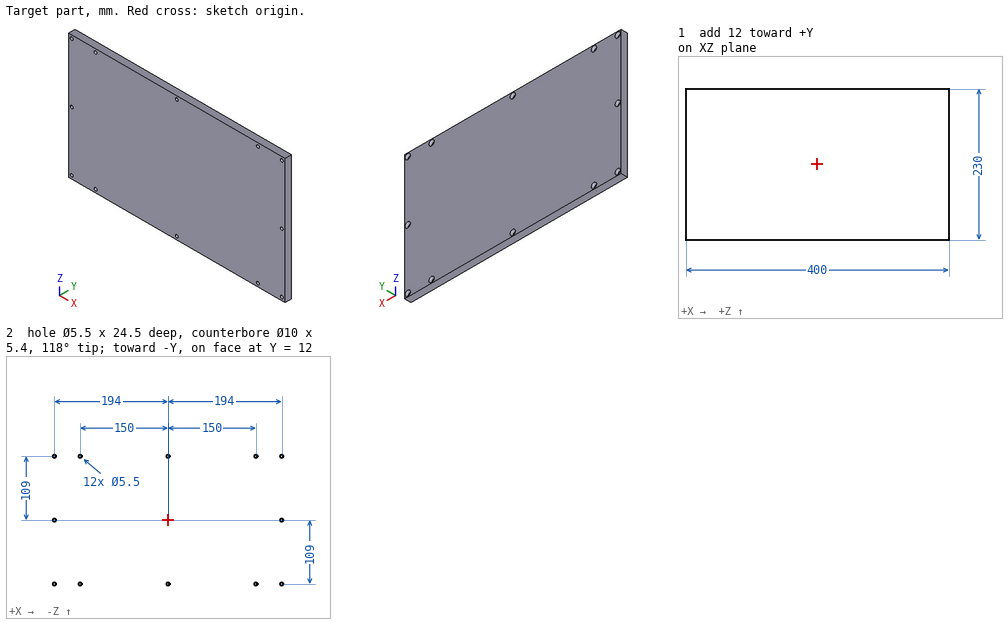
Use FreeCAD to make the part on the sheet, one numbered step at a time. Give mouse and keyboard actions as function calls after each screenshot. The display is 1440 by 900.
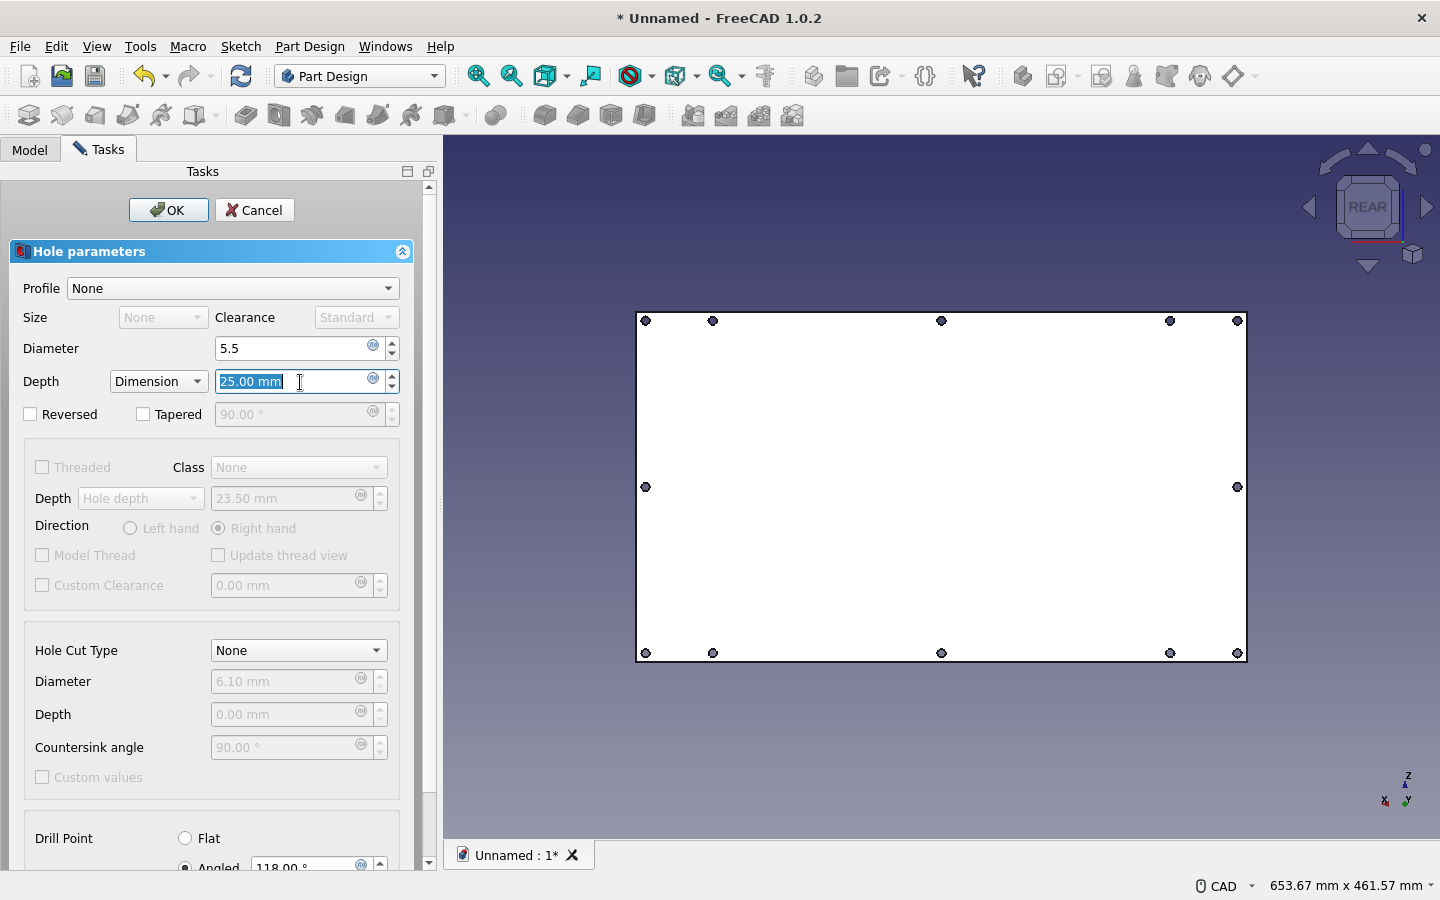
text(24.5)
key(Tab)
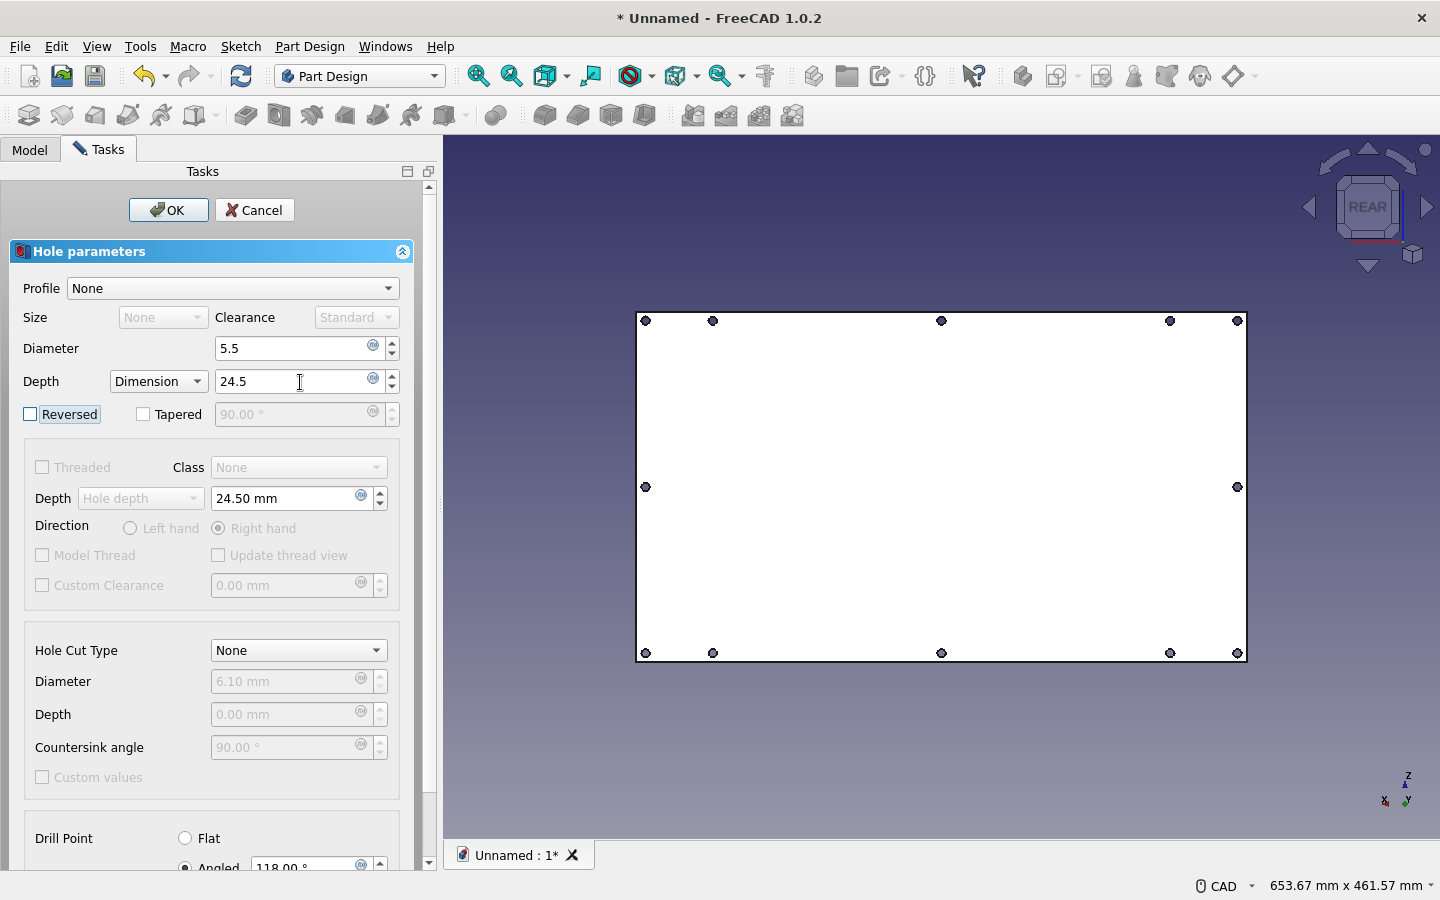
click(300, 650)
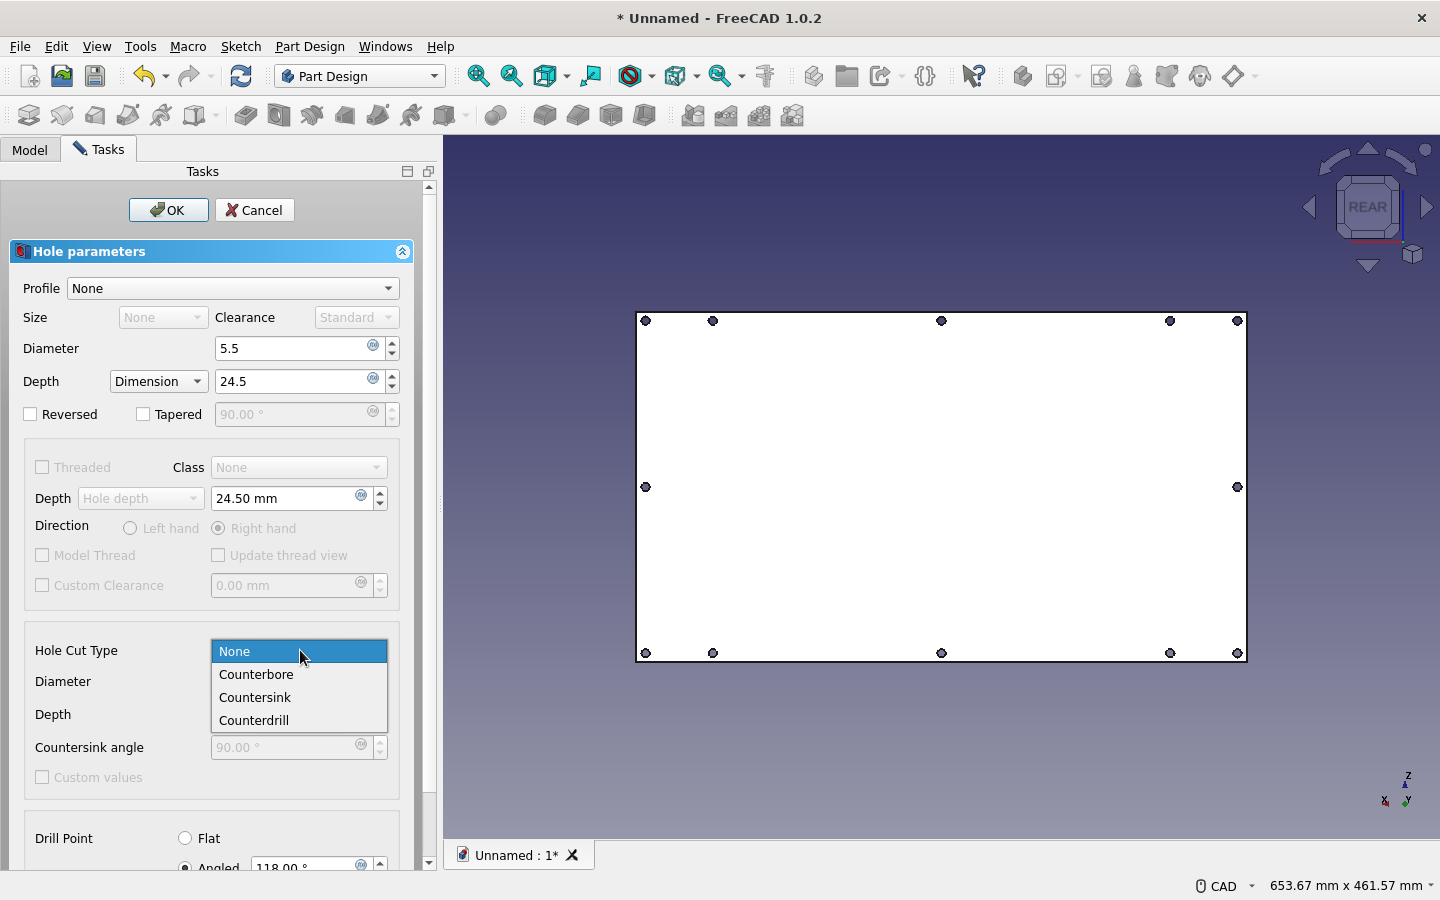
click(298, 674)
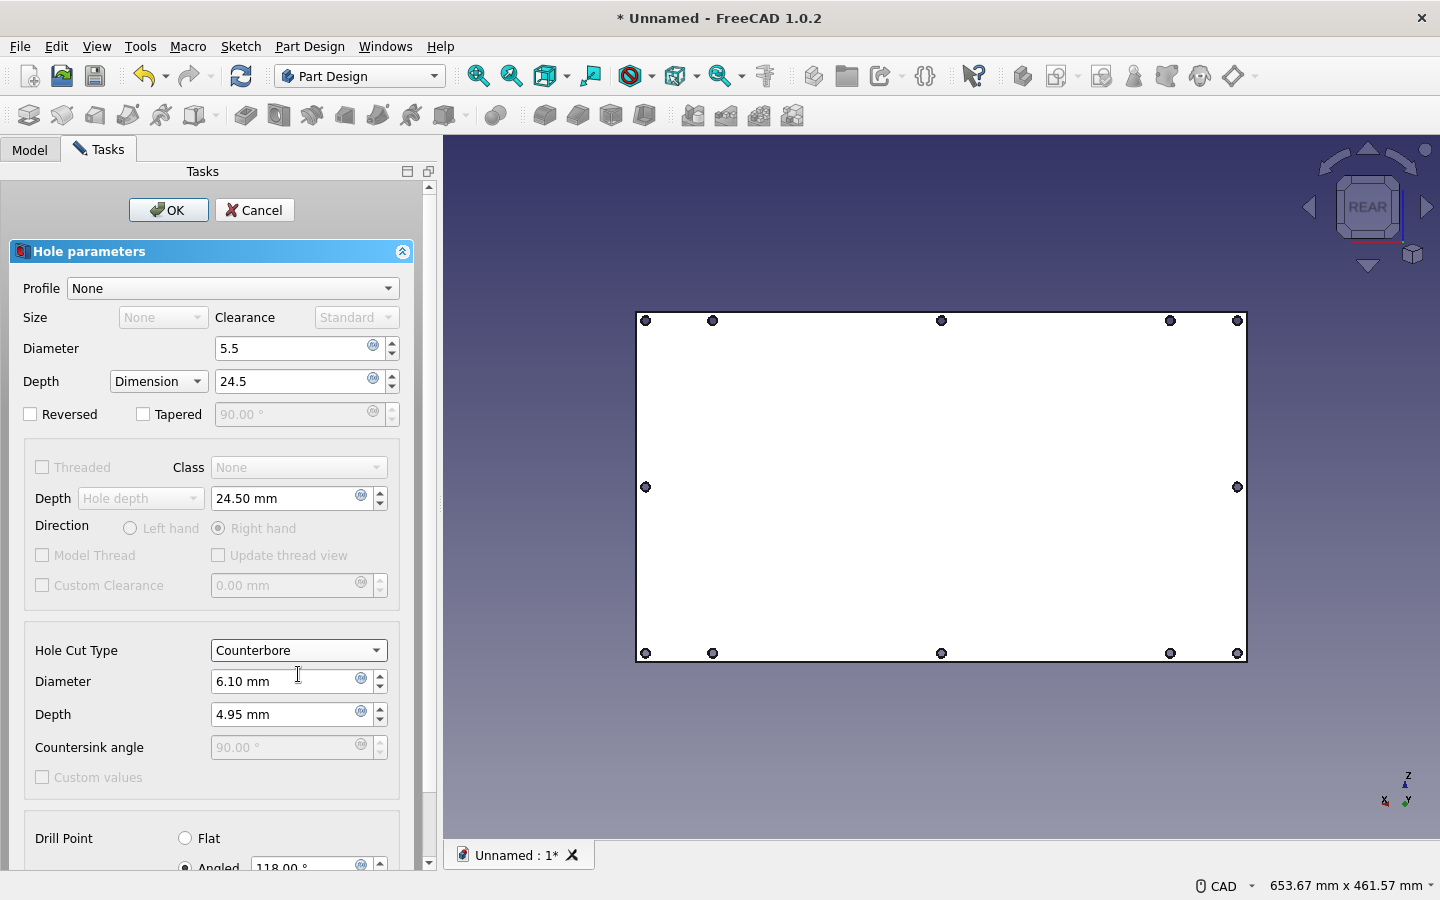
triple_click(292, 682)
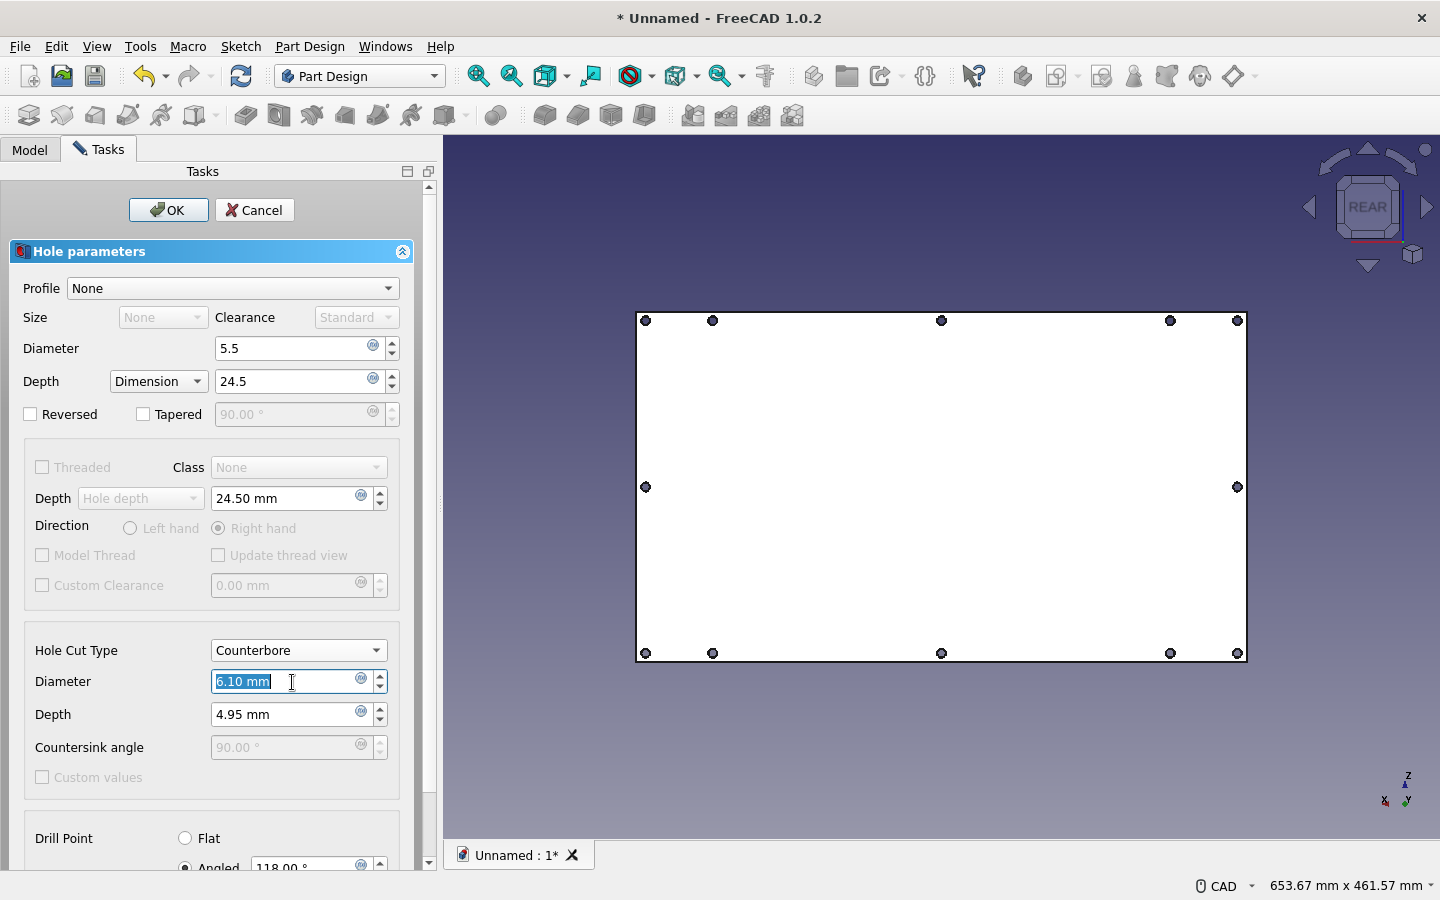
text(10)
key(Tab)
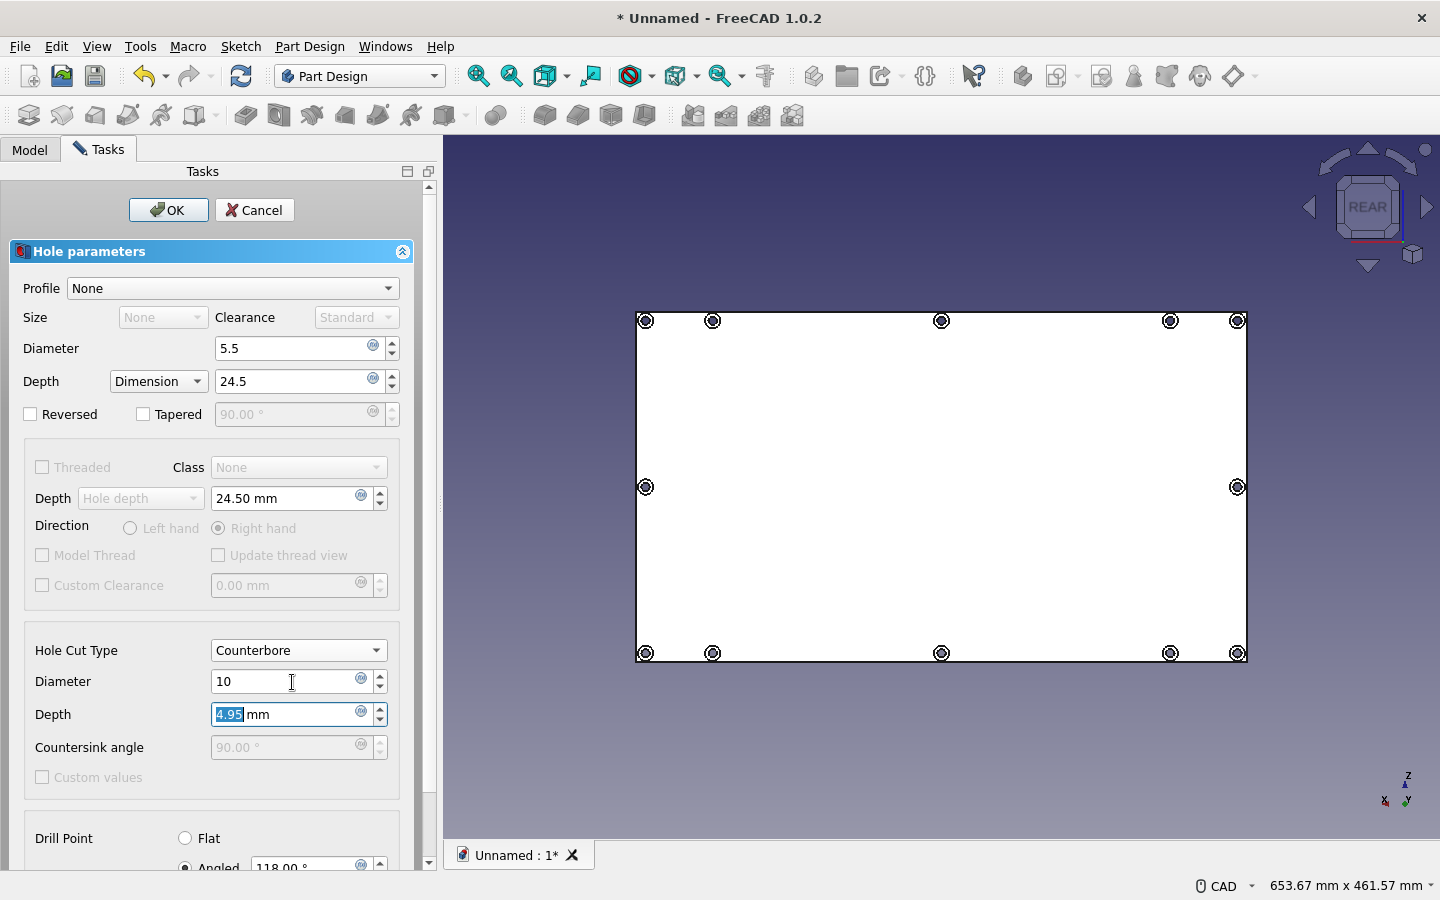
text(5.4)
key(Tab)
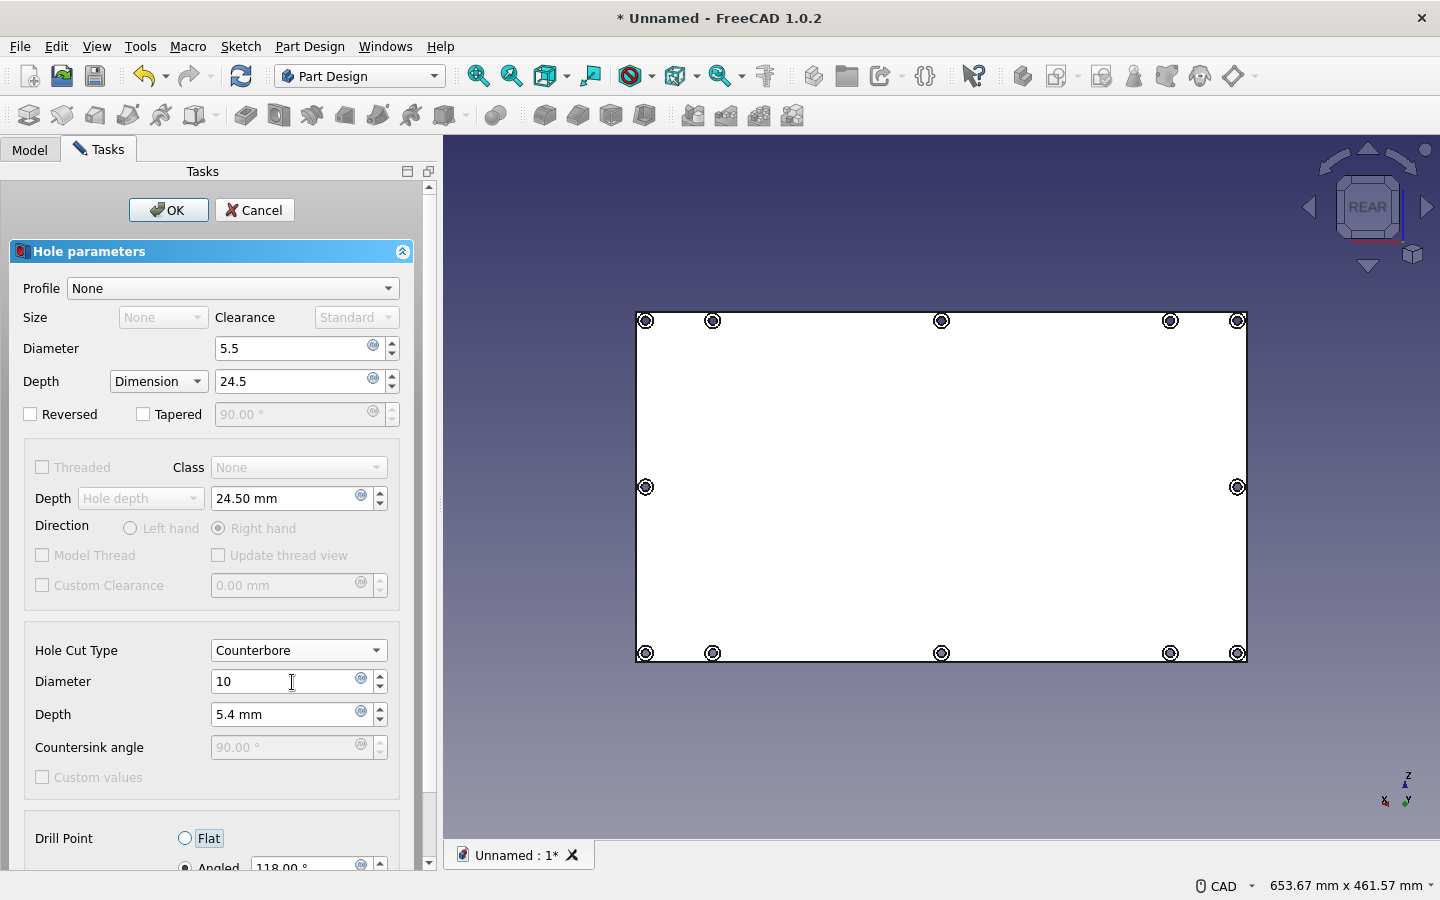
click(169, 210)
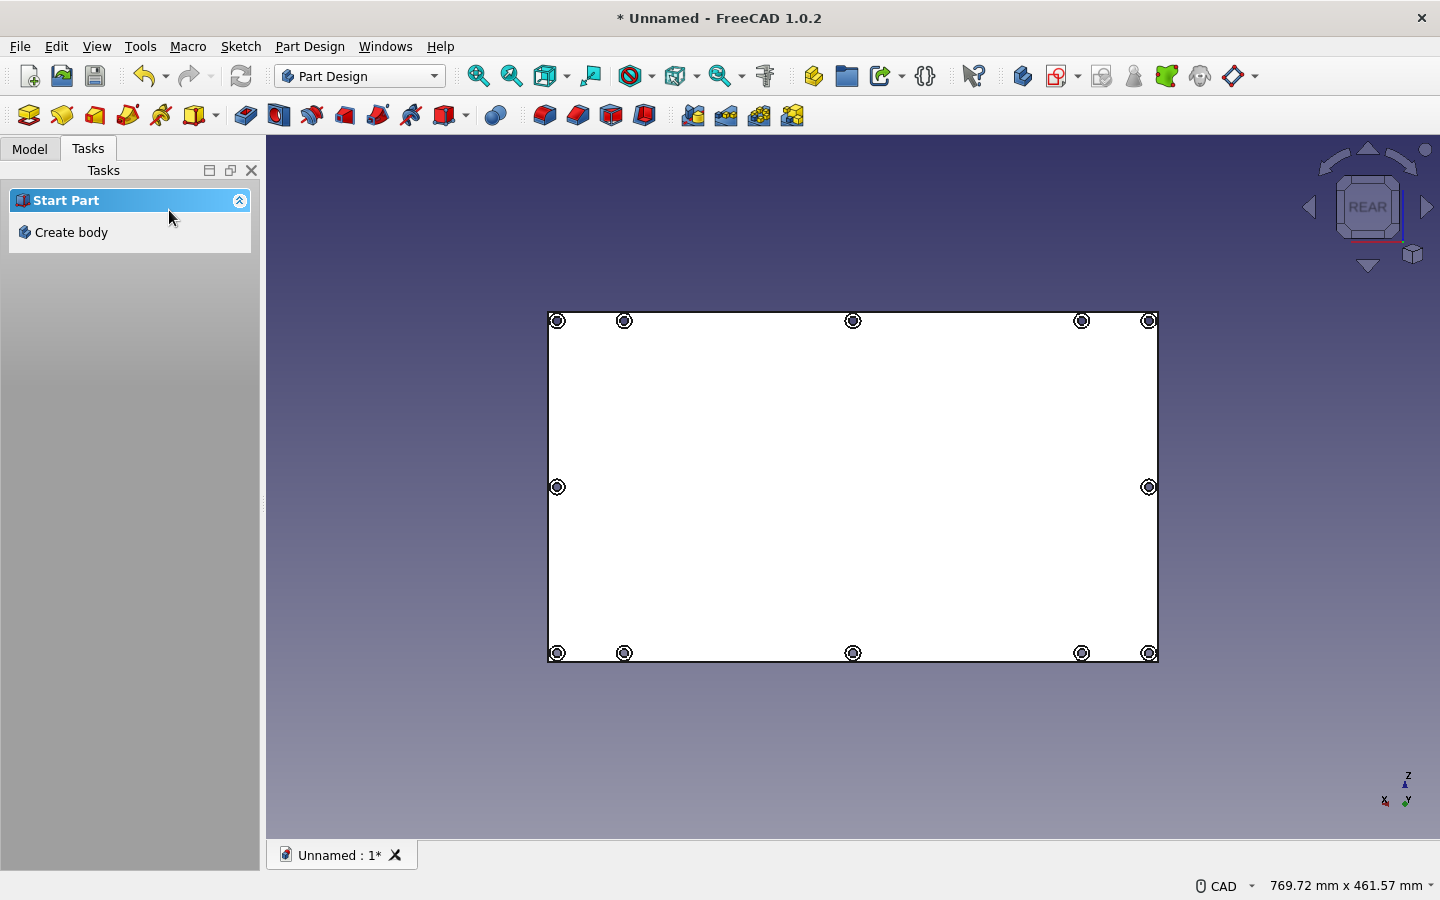
key(0)